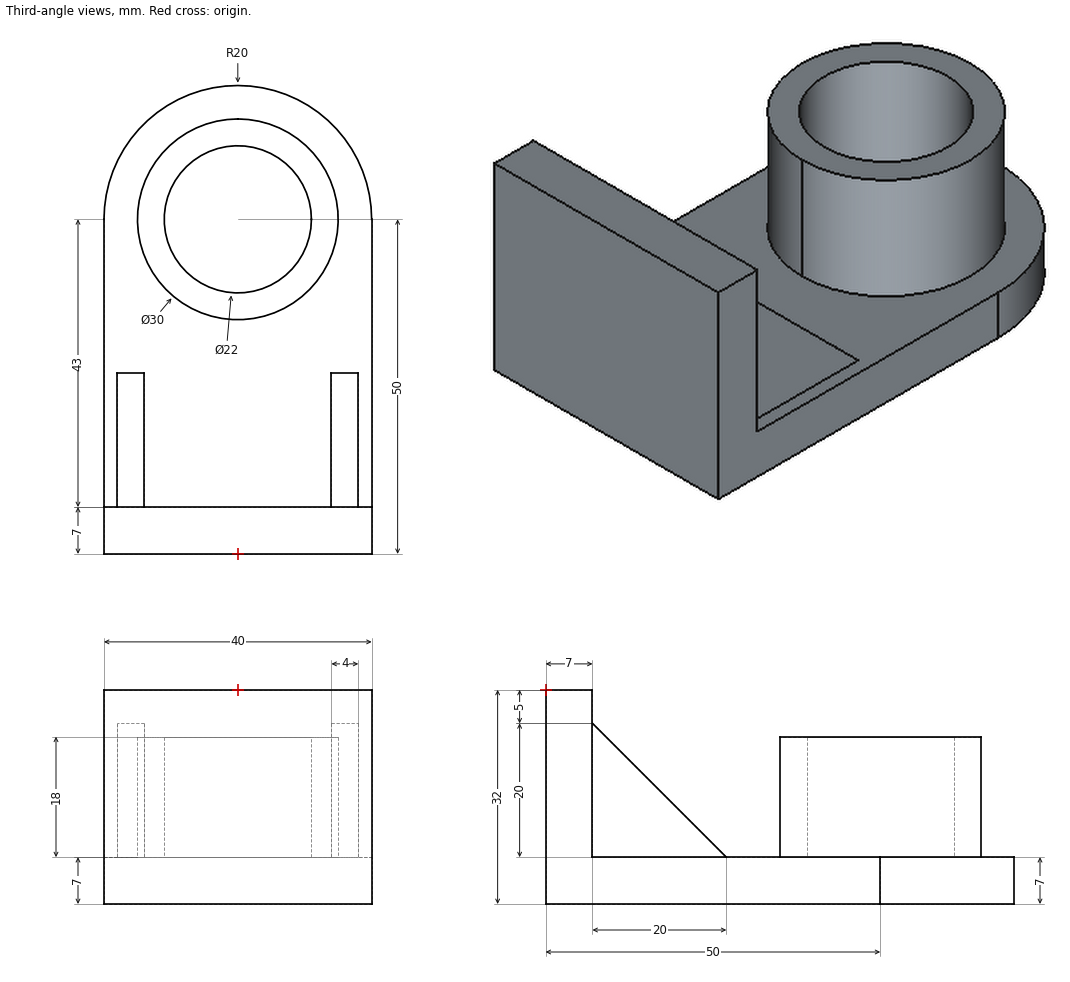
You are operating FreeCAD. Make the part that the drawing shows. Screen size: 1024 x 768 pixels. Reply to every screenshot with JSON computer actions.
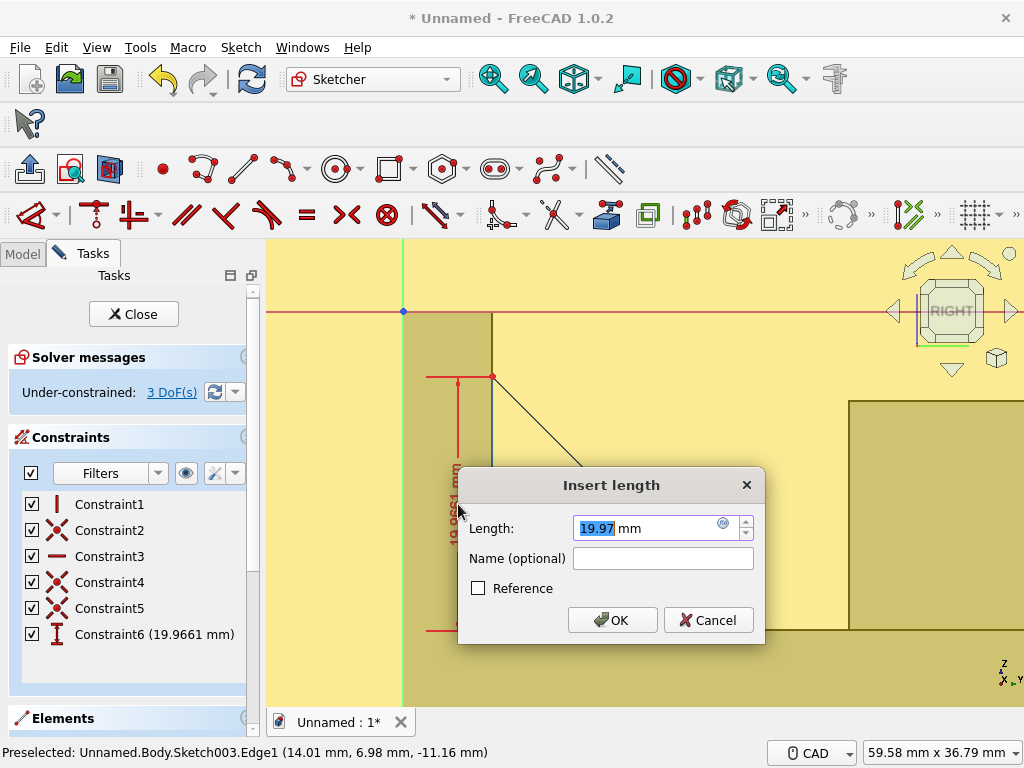
{"action": "type", "text": "20"}
{"action": "key", "text": "Return"}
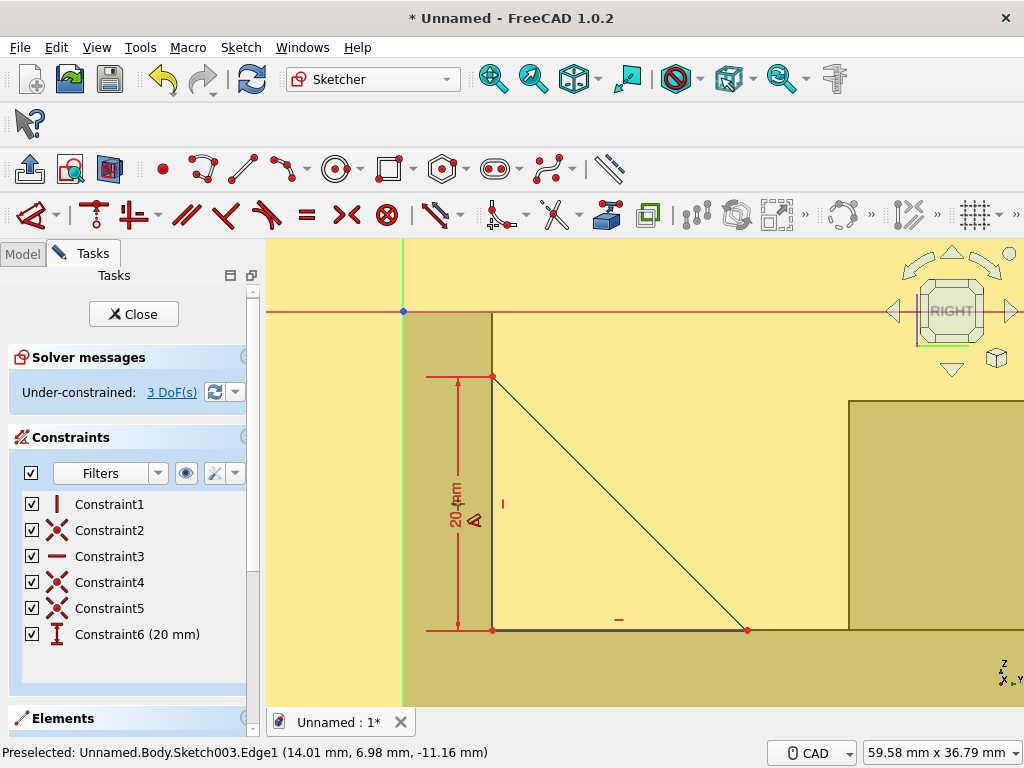
{"action": "left_click", "coordinate": [569, 631]}
{"action": "left_click", "coordinate": [619, 665]}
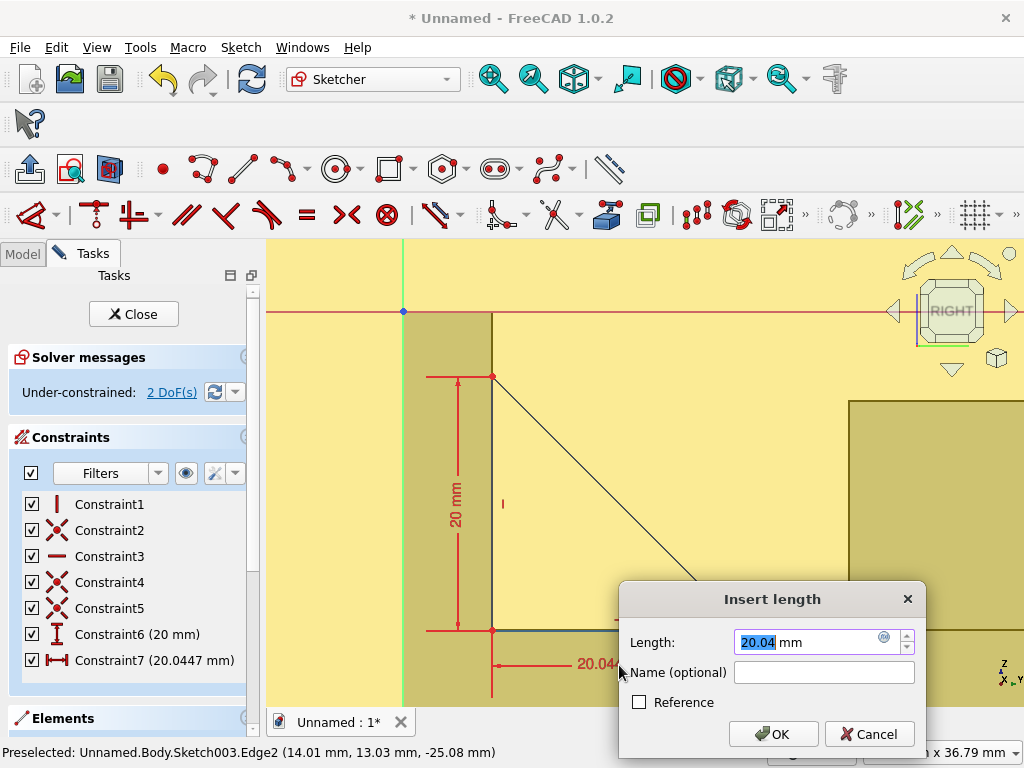
{"action": "type", "text": "20"}
{"action": "key", "text": "Return"}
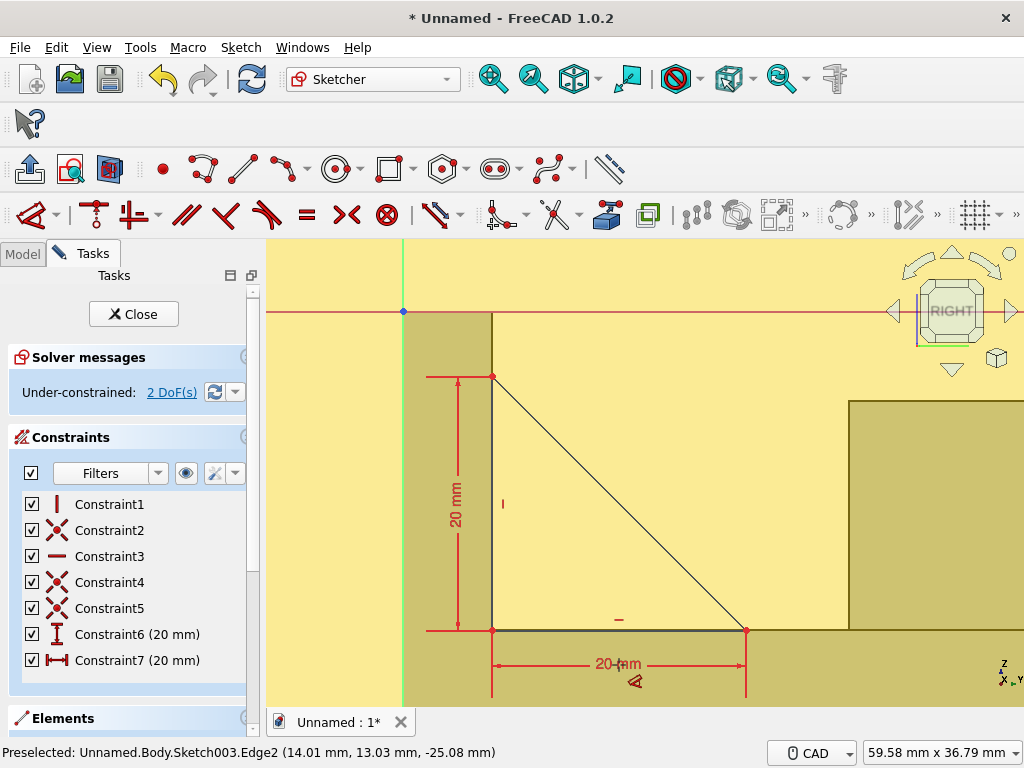
{"action": "left_click", "coordinate": [492, 377]}
{"action": "left_click", "coordinate": [448, 278]}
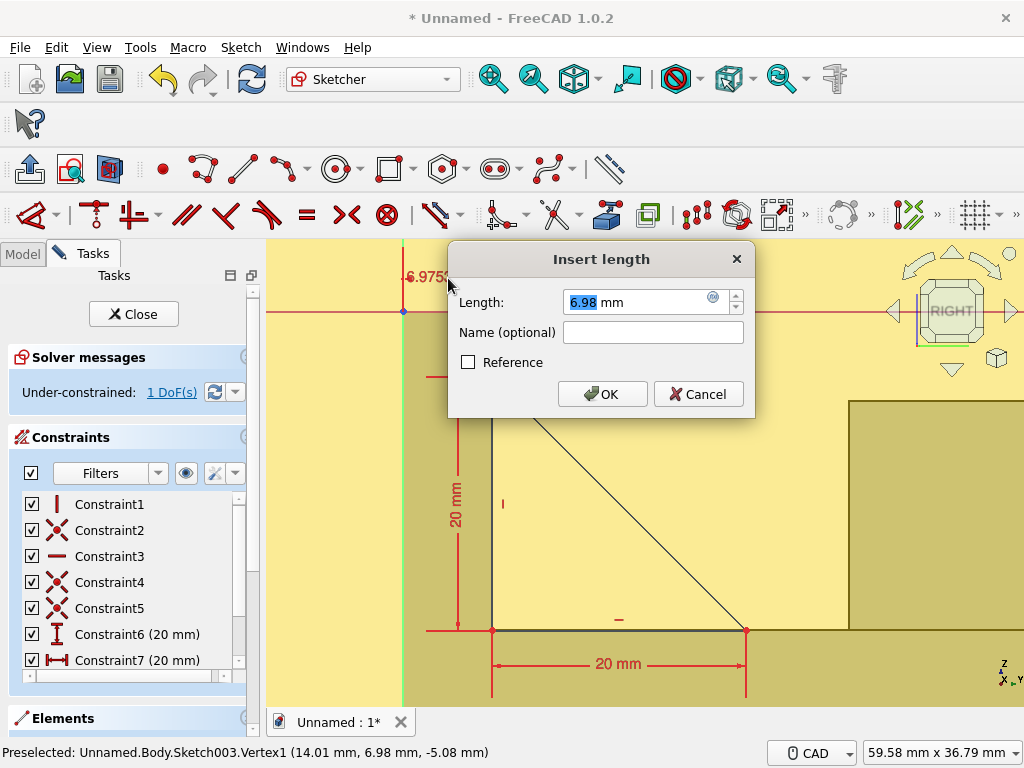
{"action": "type", "text": "7"}
{"action": "key", "text": "Return"}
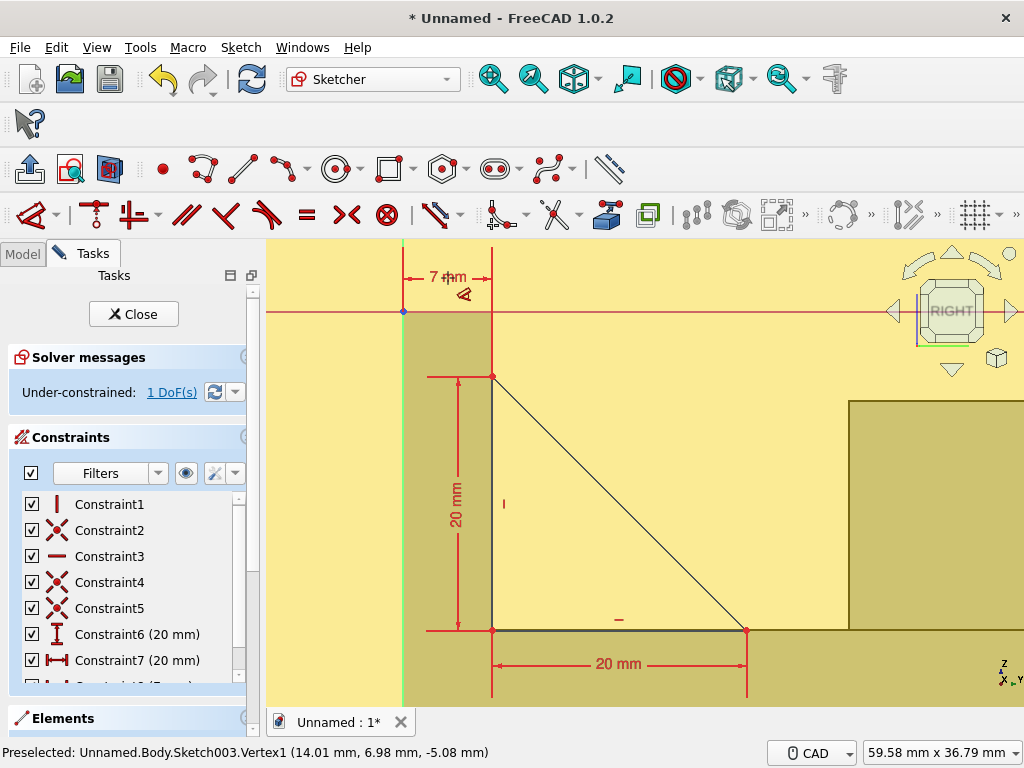
{"action": "left_click", "coordinate": [492, 377]}
{"action": "left_click", "coordinate": [369, 344]}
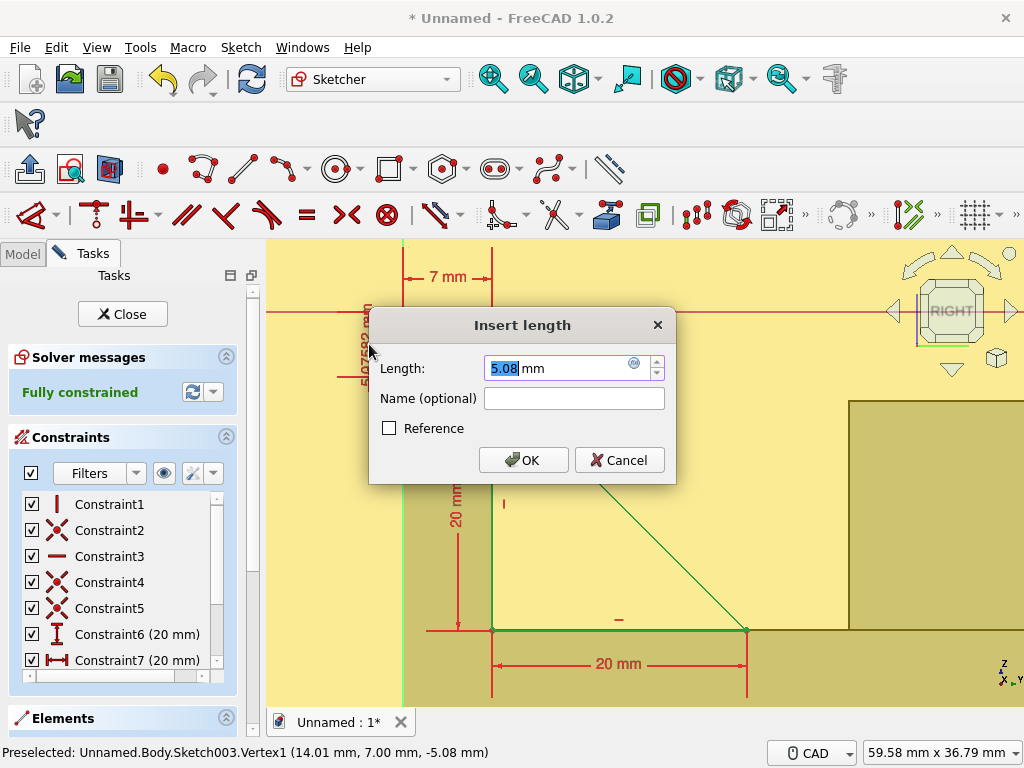
{"action": "type", "text": "5"}
{"action": "key", "text": "Return"}
{"action": "key", "text": "Escape"}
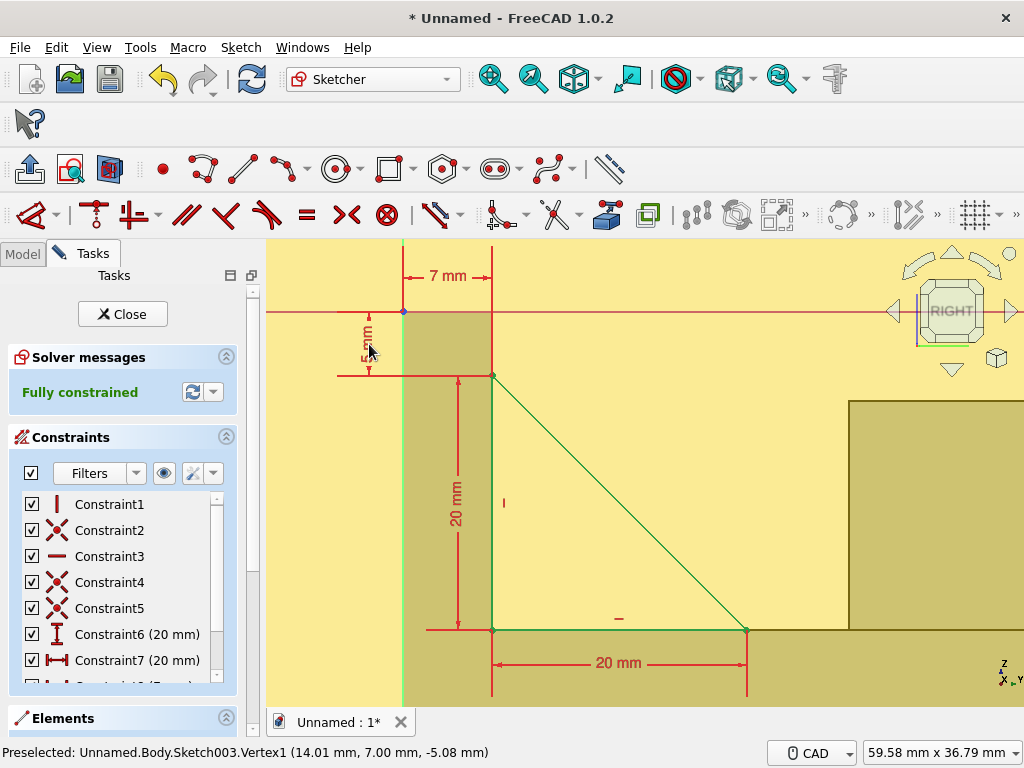
{"action": "left_click", "coordinate": [123, 314]}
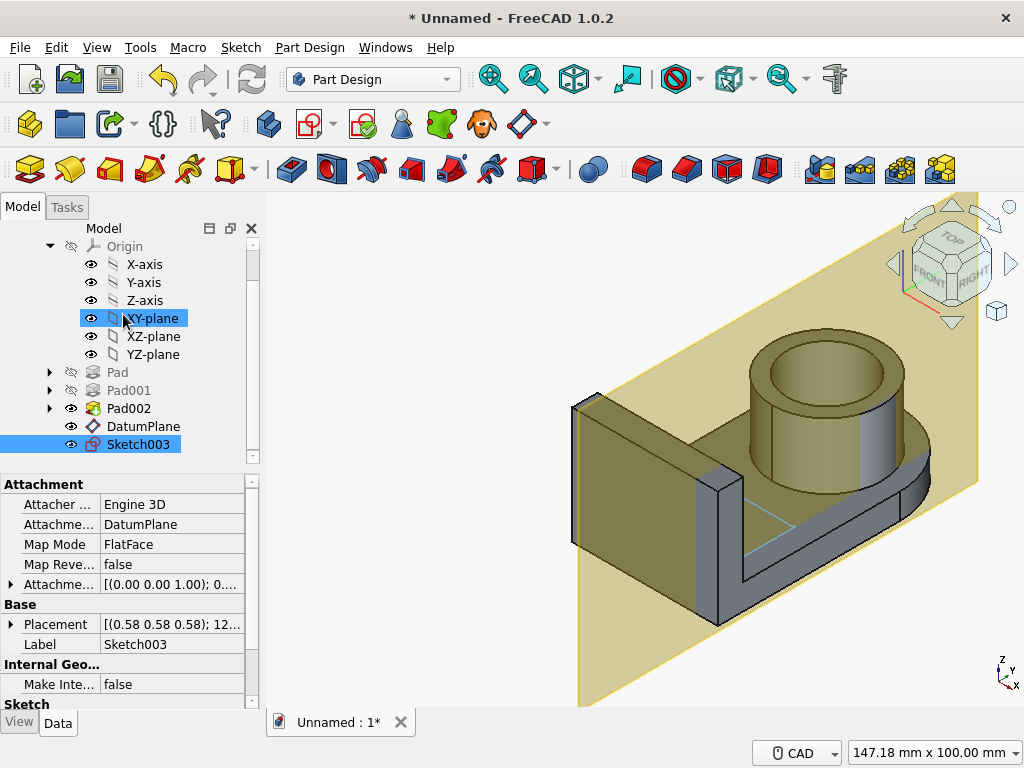
{"action": "left_click", "coordinate": [30, 170]}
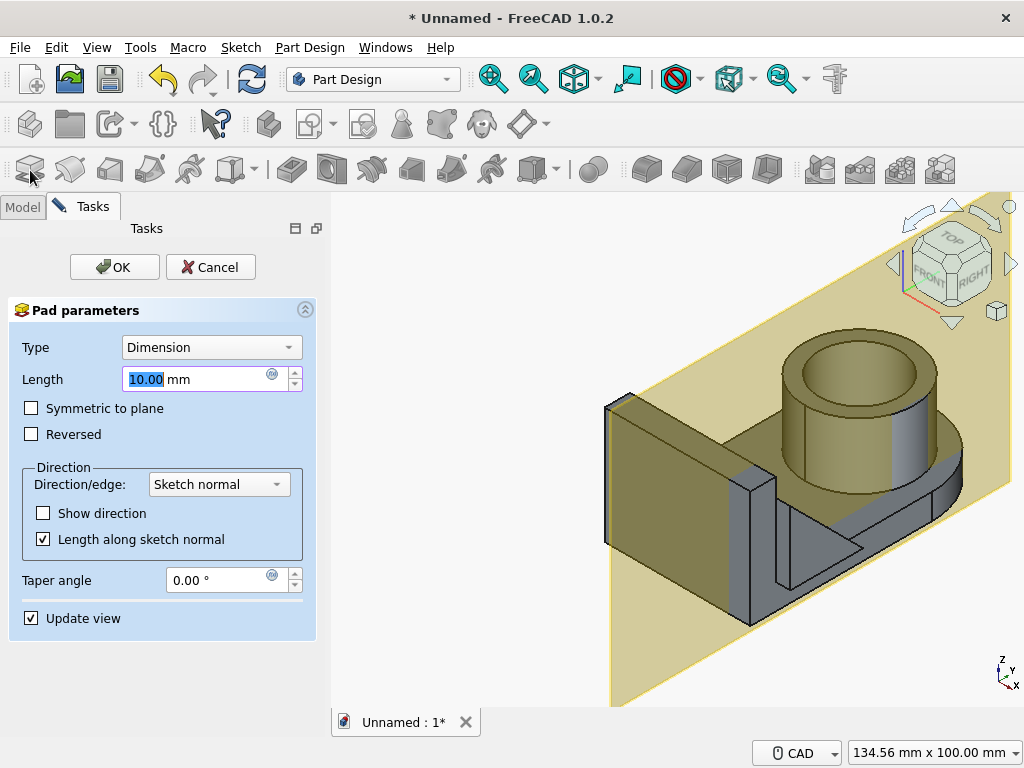
{"action": "type", "text": "4"}
{"action": "key", "text": "Tab"}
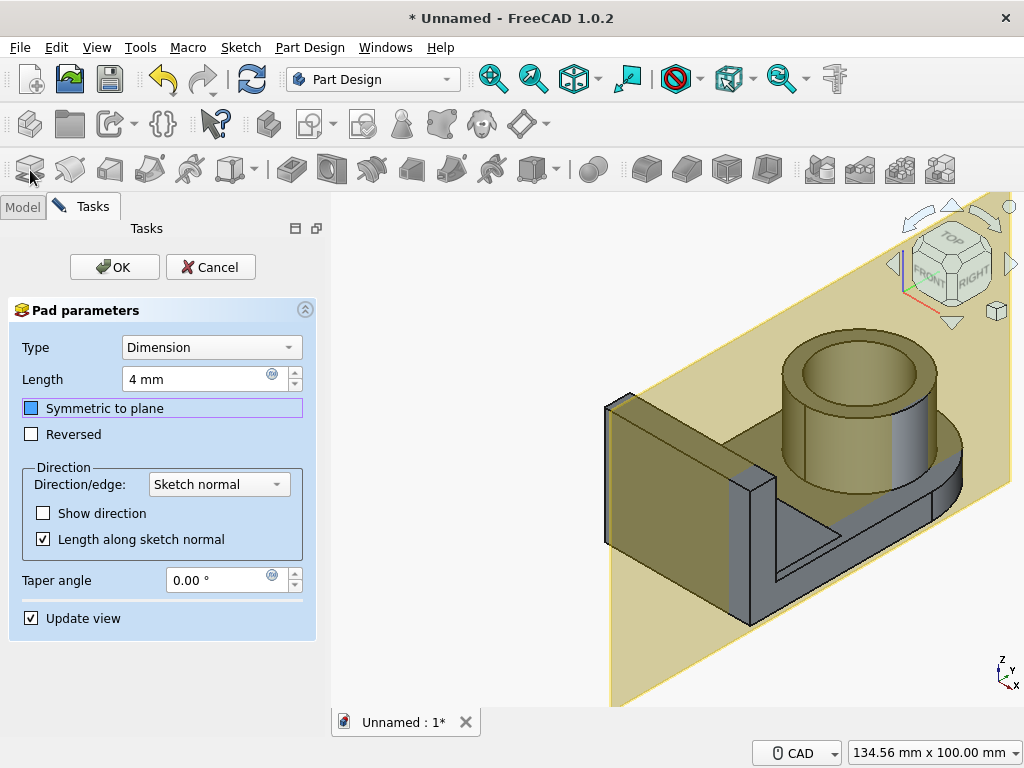
{"action": "left_click", "coordinate": [115, 267]}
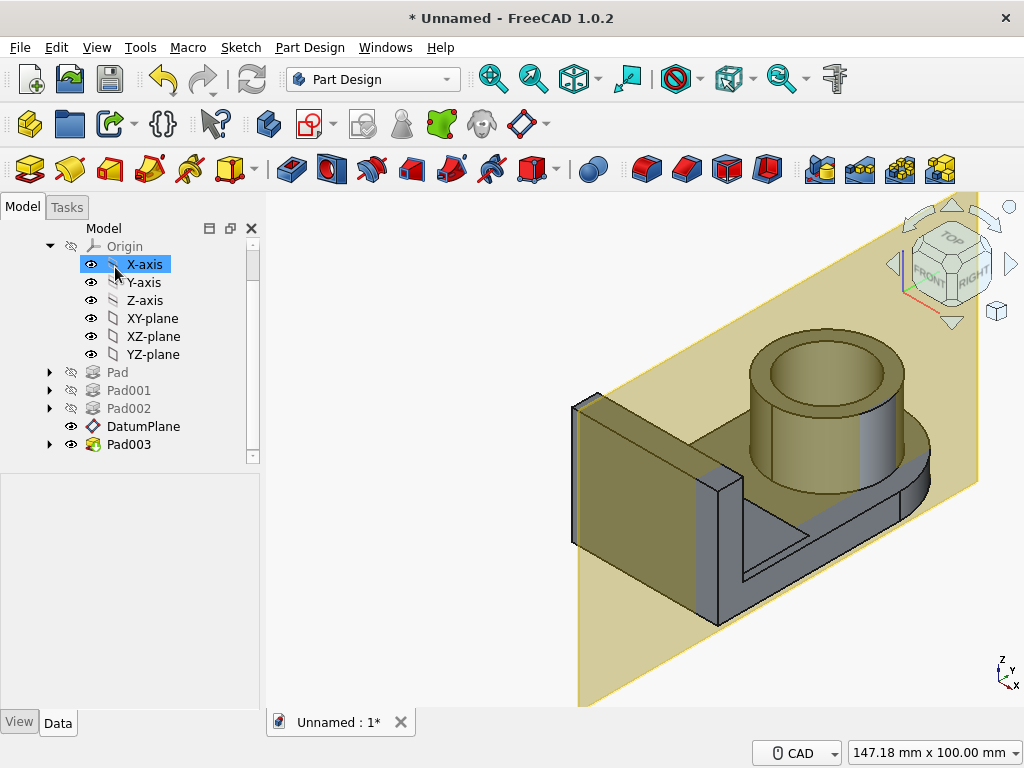
{"action": "left_click", "coordinate": [116, 426]}
{"action": "key", "text": "space"}